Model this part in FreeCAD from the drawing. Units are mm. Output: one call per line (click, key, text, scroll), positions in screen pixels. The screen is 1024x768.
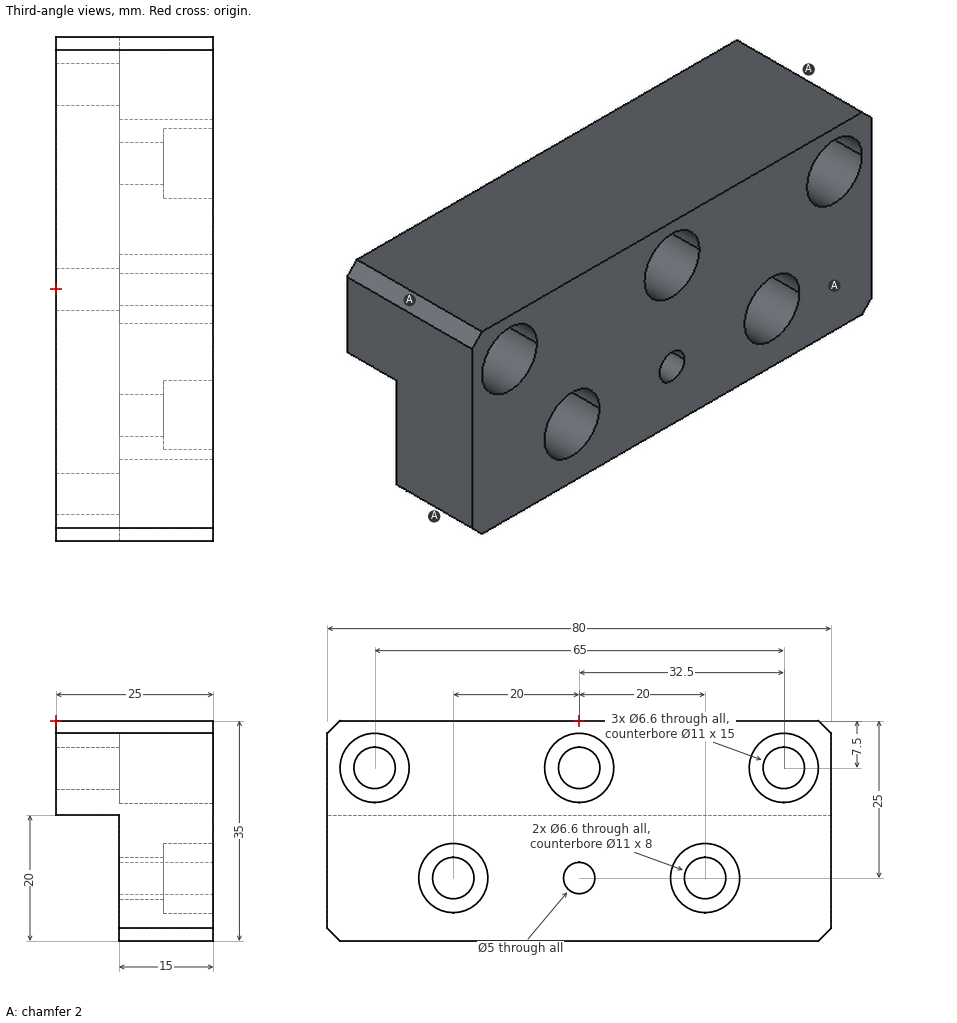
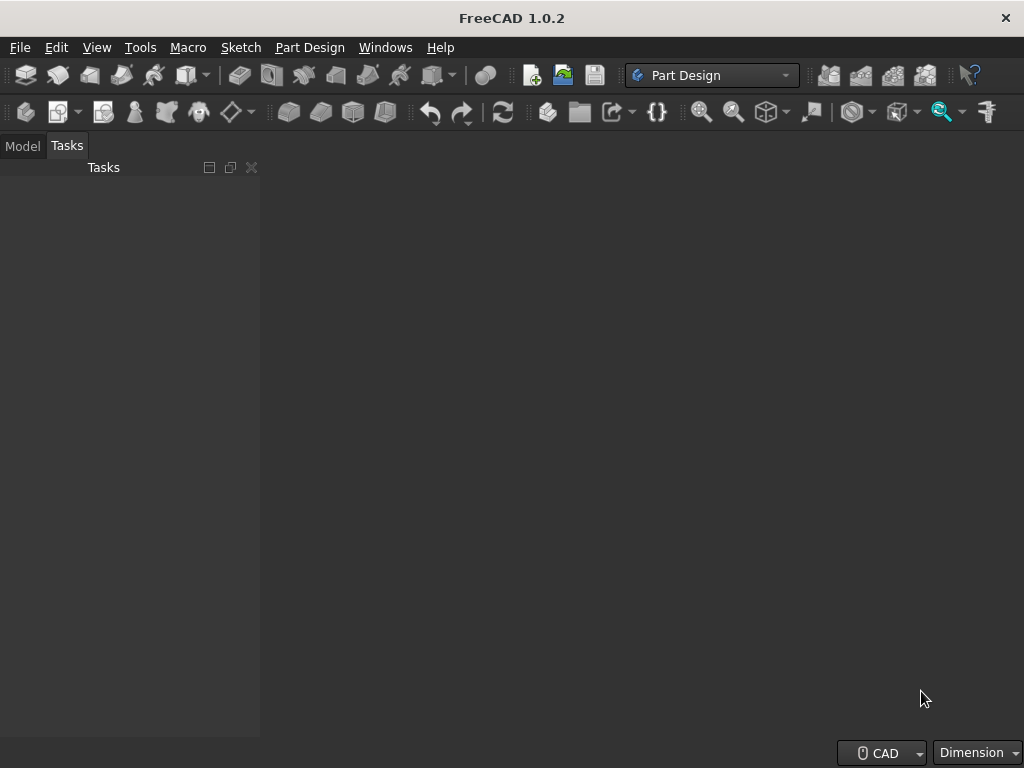
click(532, 76)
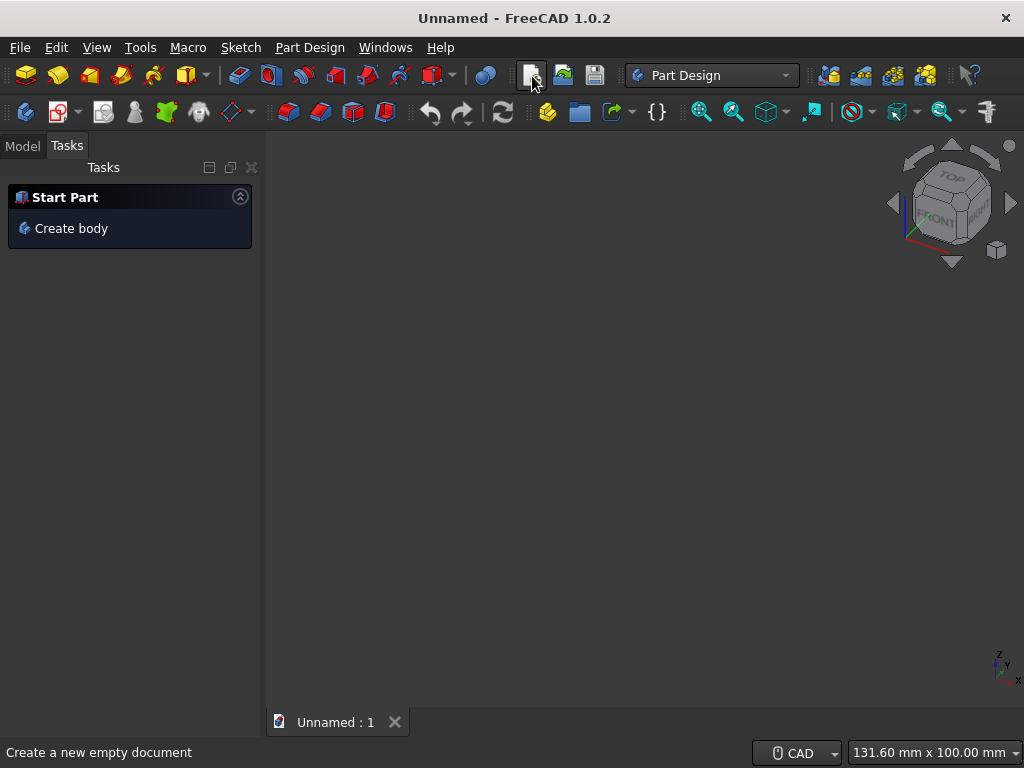
click(58, 112)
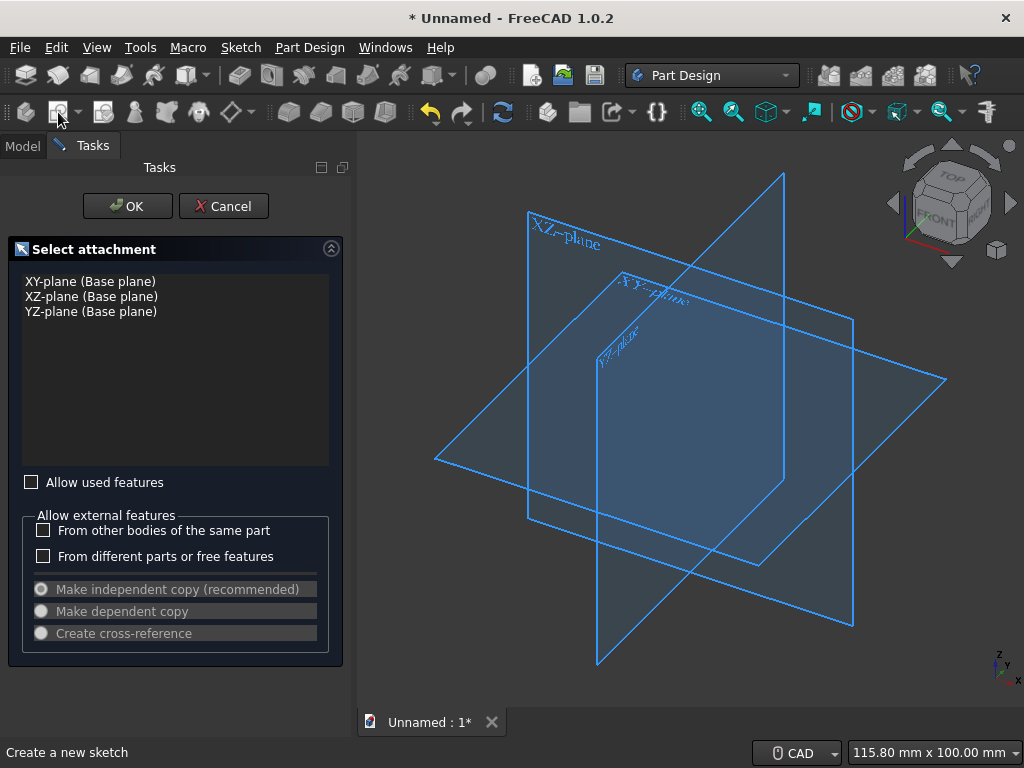
click(82, 296)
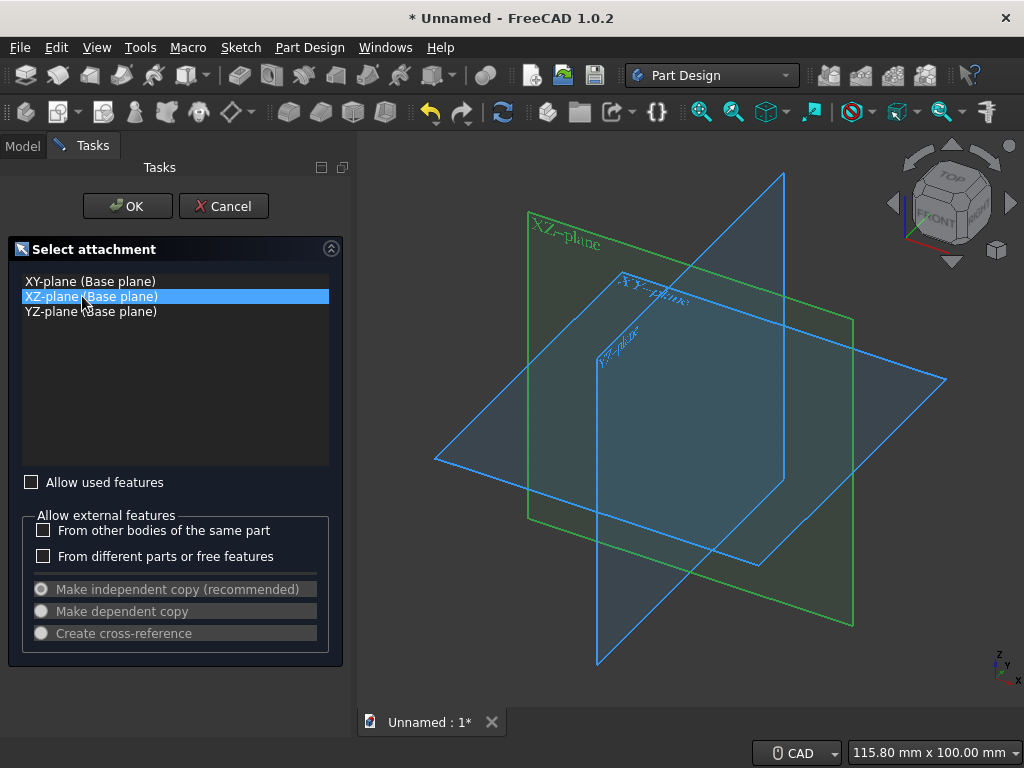
click(128, 206)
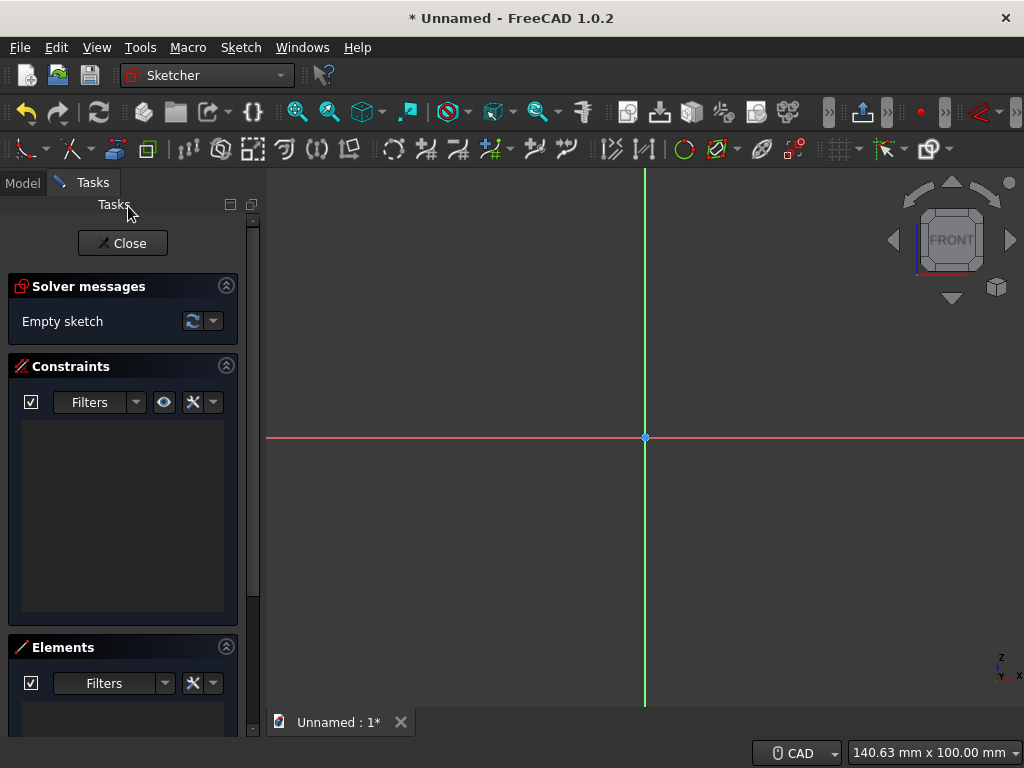
scroll(859, 647, up, 3)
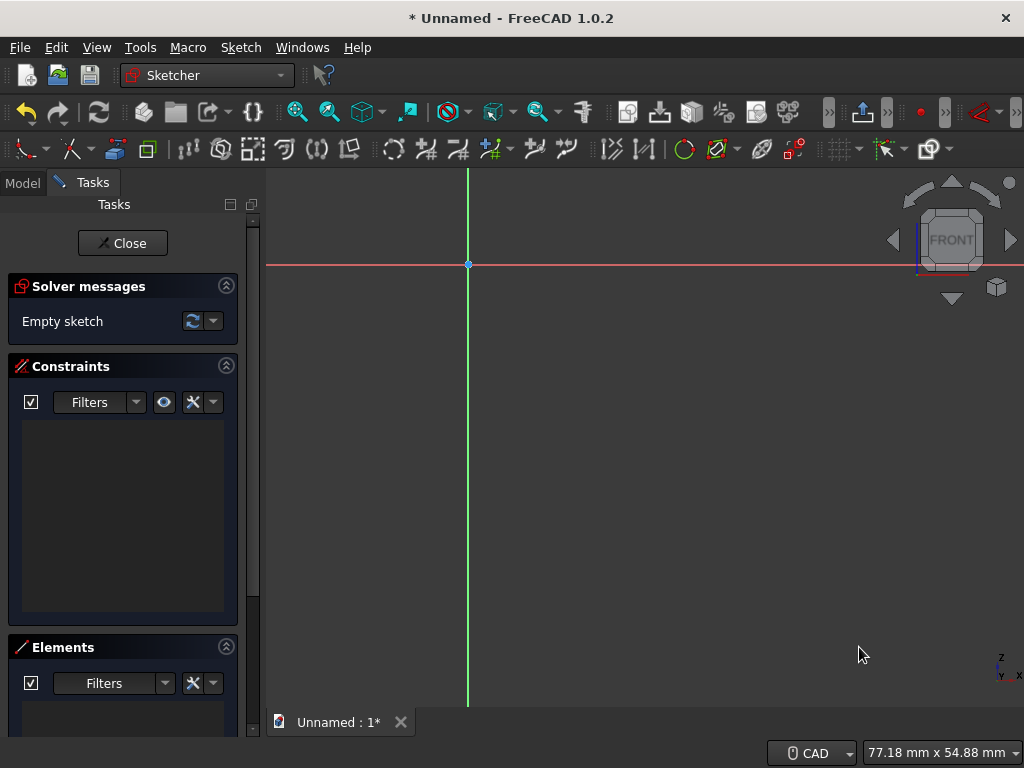
key(g)
key(m)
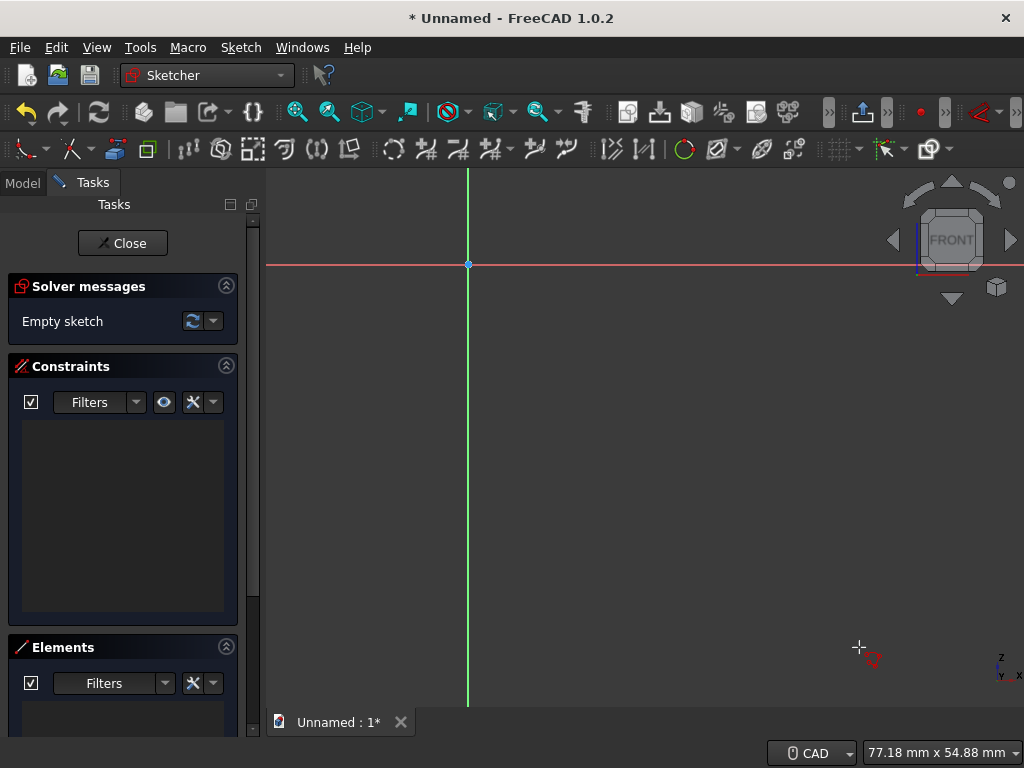
click(468, 265)
click(714, 274)
click(714, 608)
click(567, 608)
click(567, 412)
click(477, 412)
click(468, 265)
key(Escape)
key(Escape)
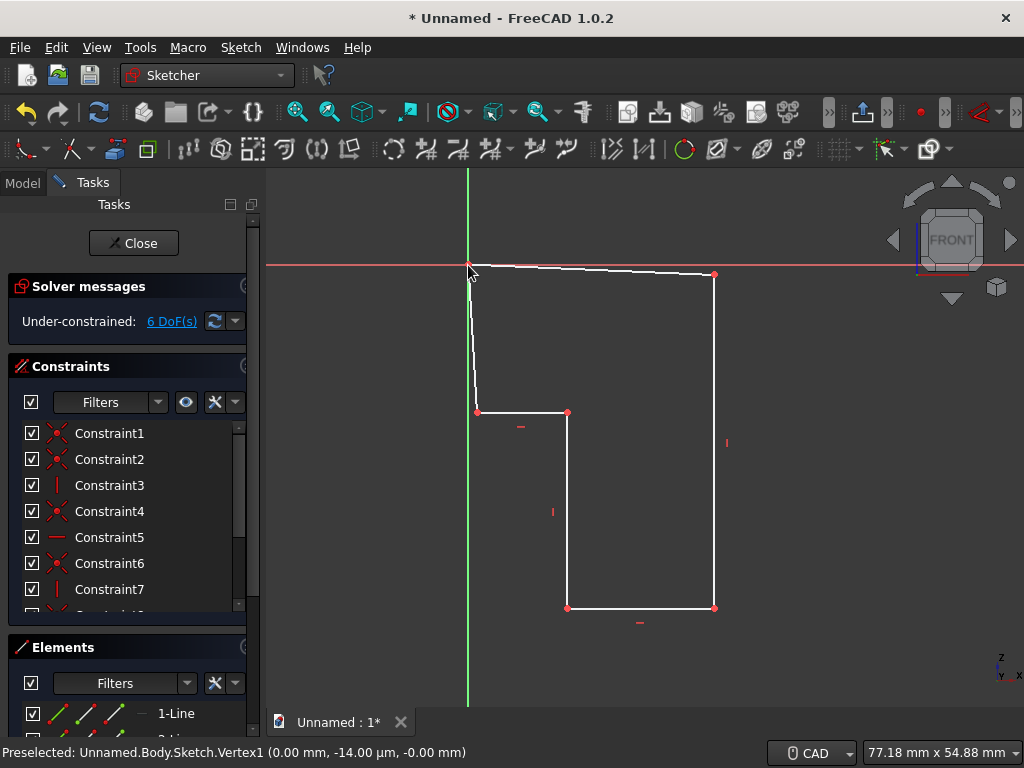
click(542, 268)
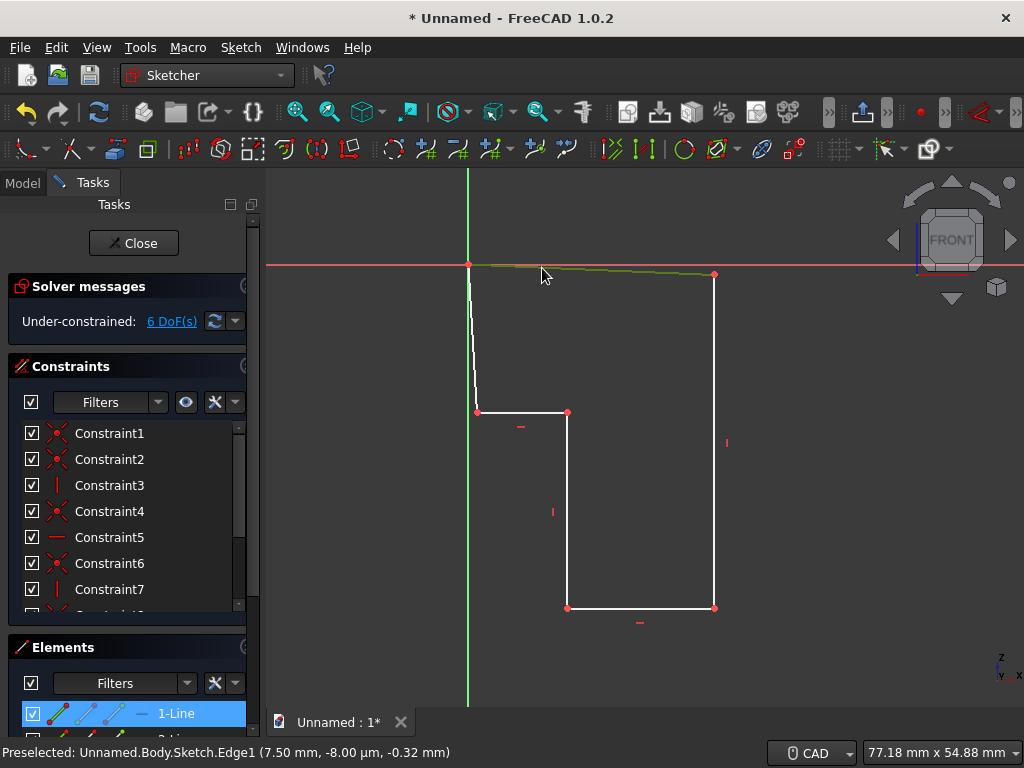
key(h)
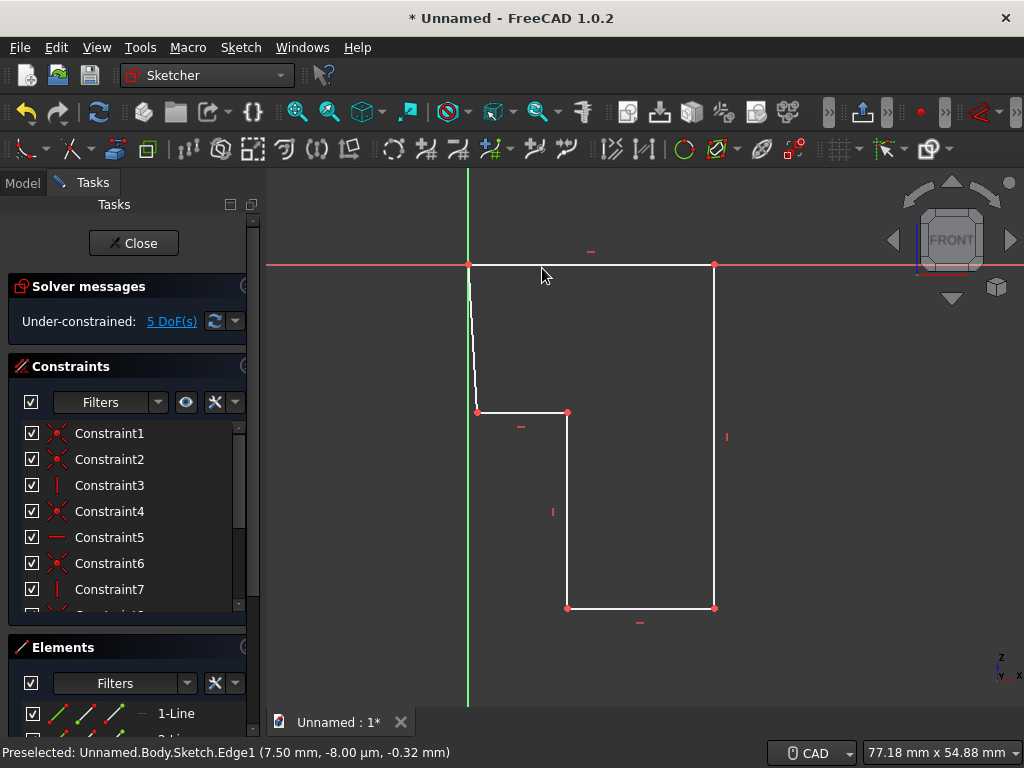
click(471, 309)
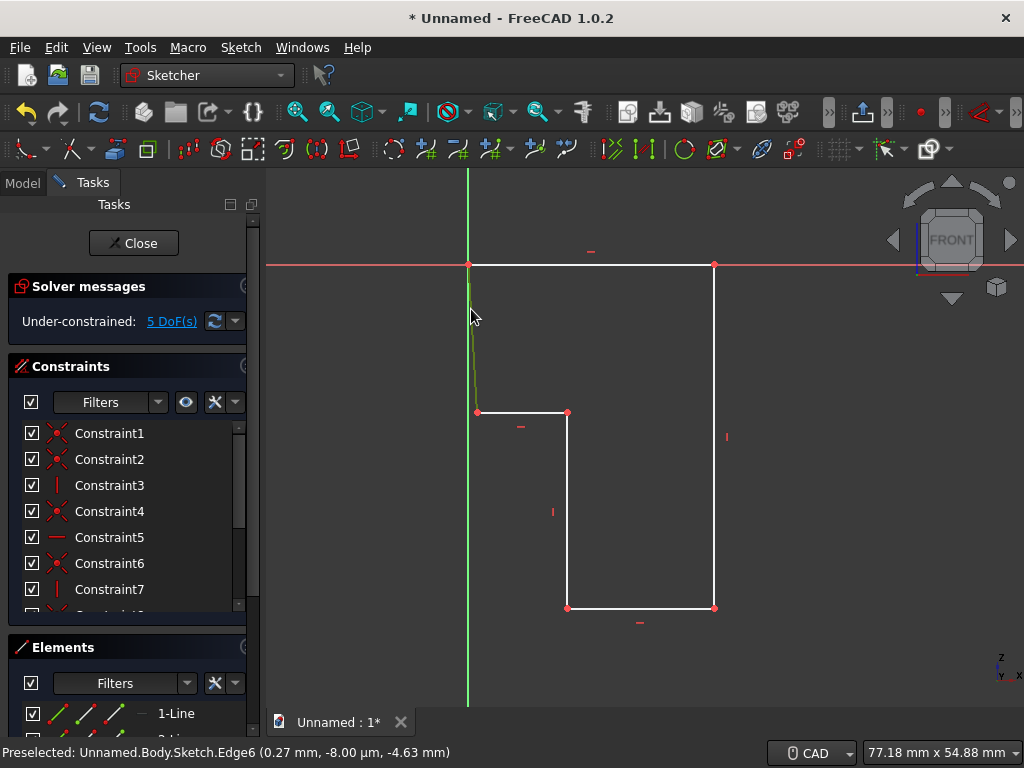
key(v)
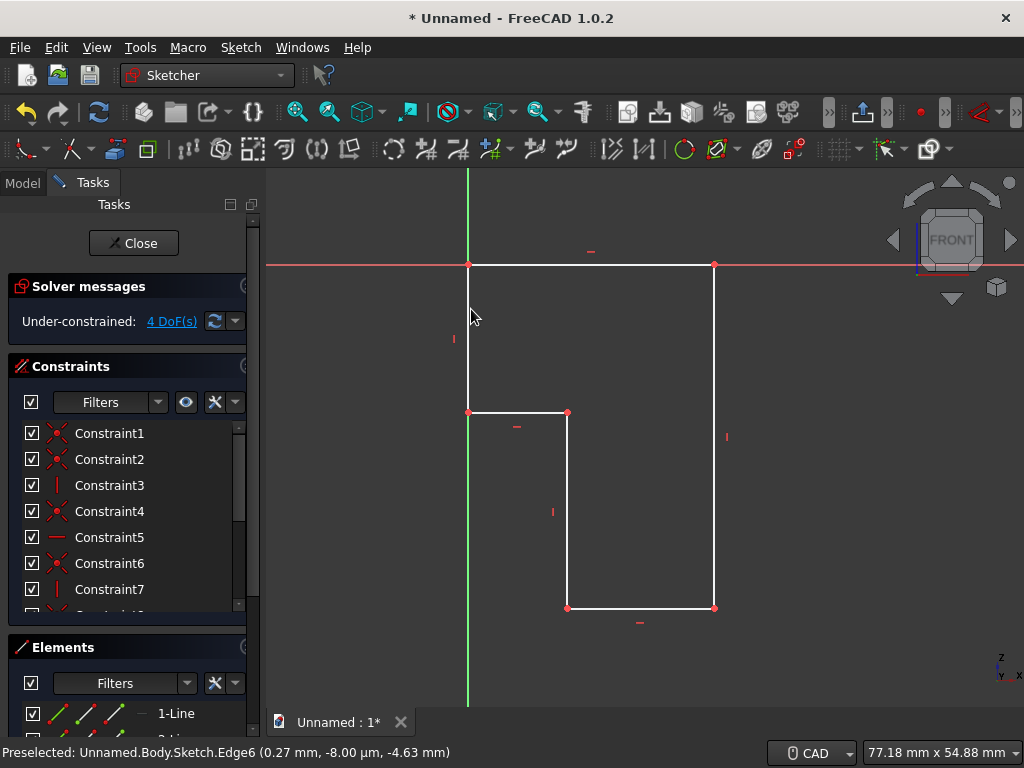
click(980, 112)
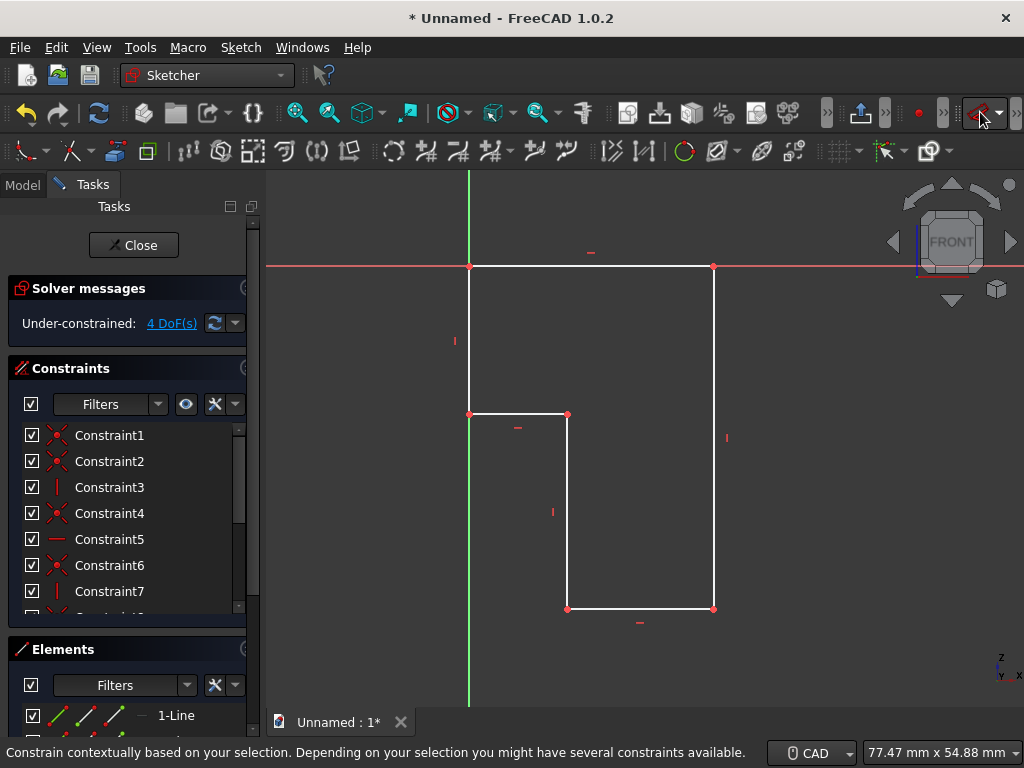
click(542, 266)
click(591, 232)